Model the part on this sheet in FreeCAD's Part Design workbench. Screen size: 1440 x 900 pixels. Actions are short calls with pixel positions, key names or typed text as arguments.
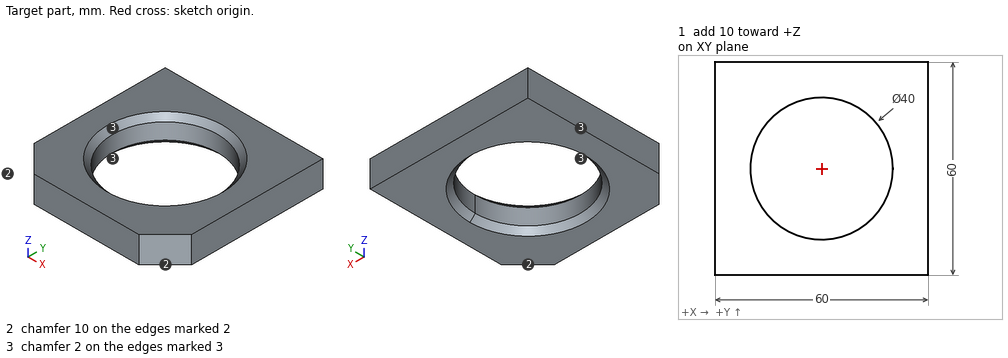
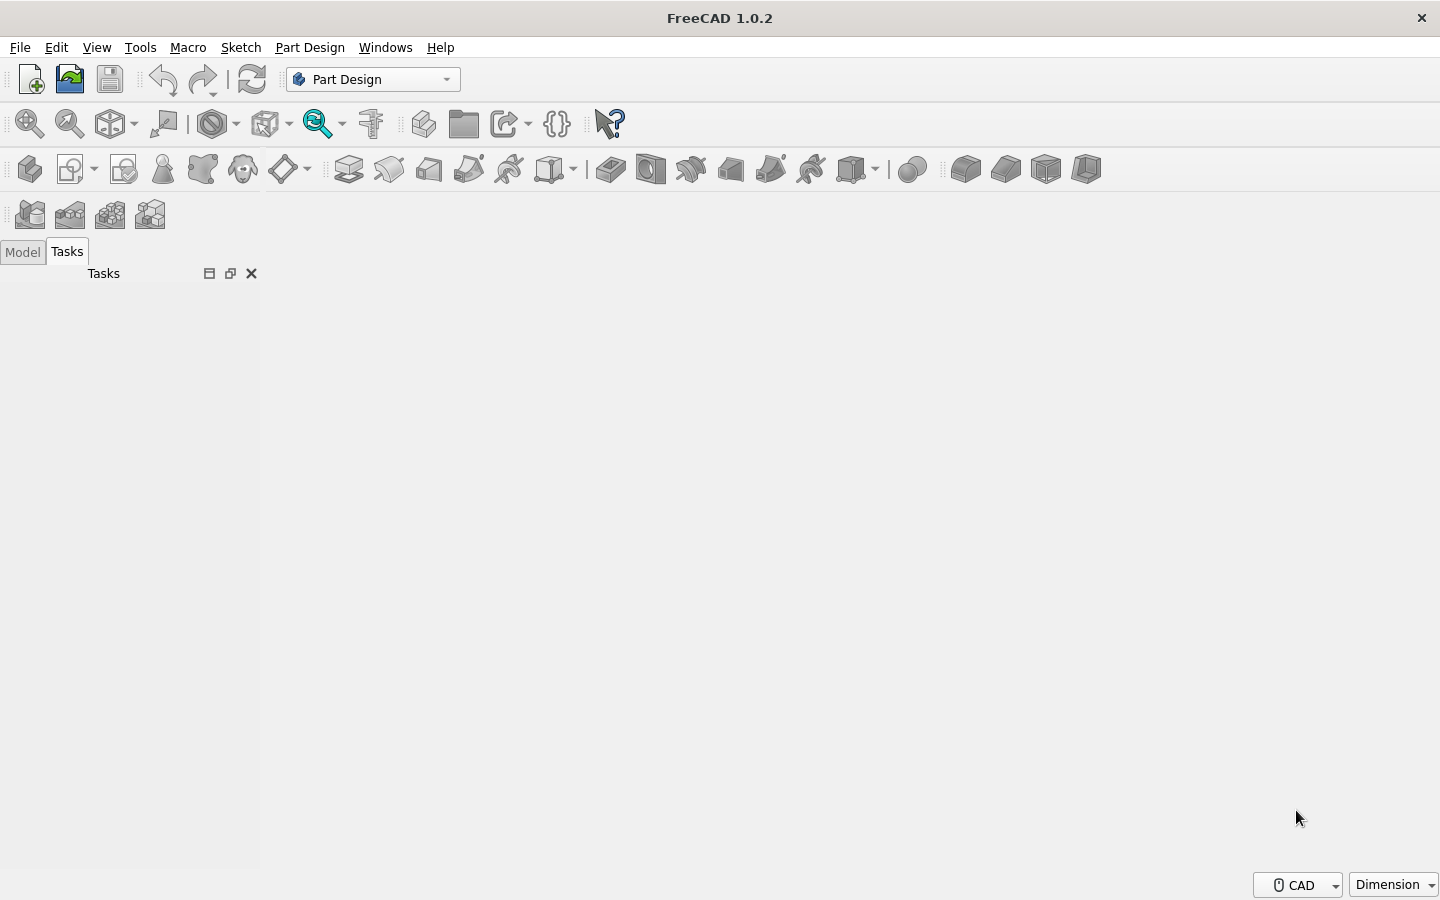
click(584, 80)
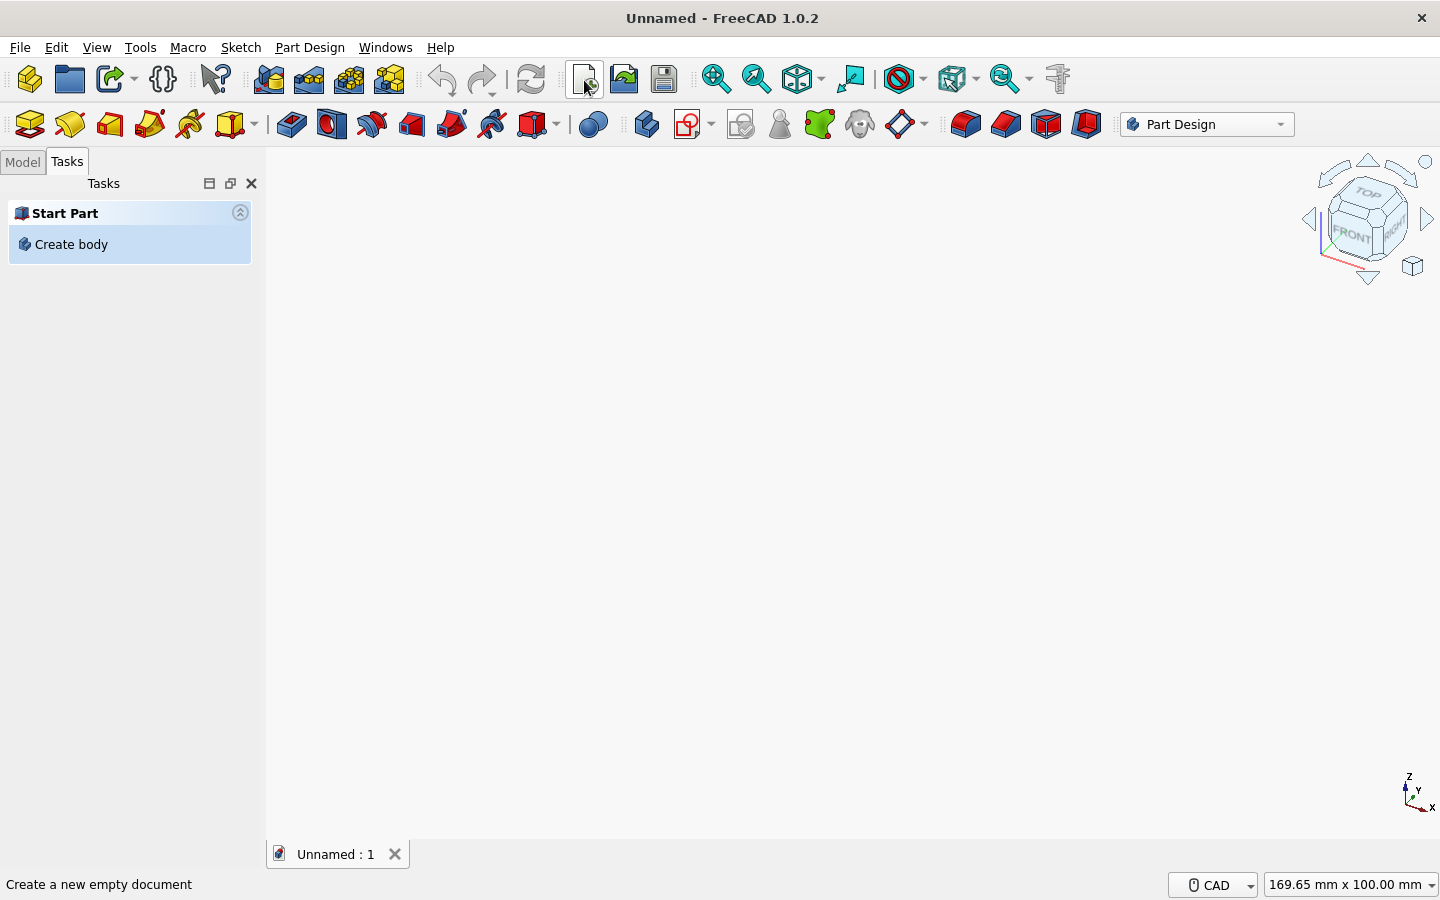
click(688, 124)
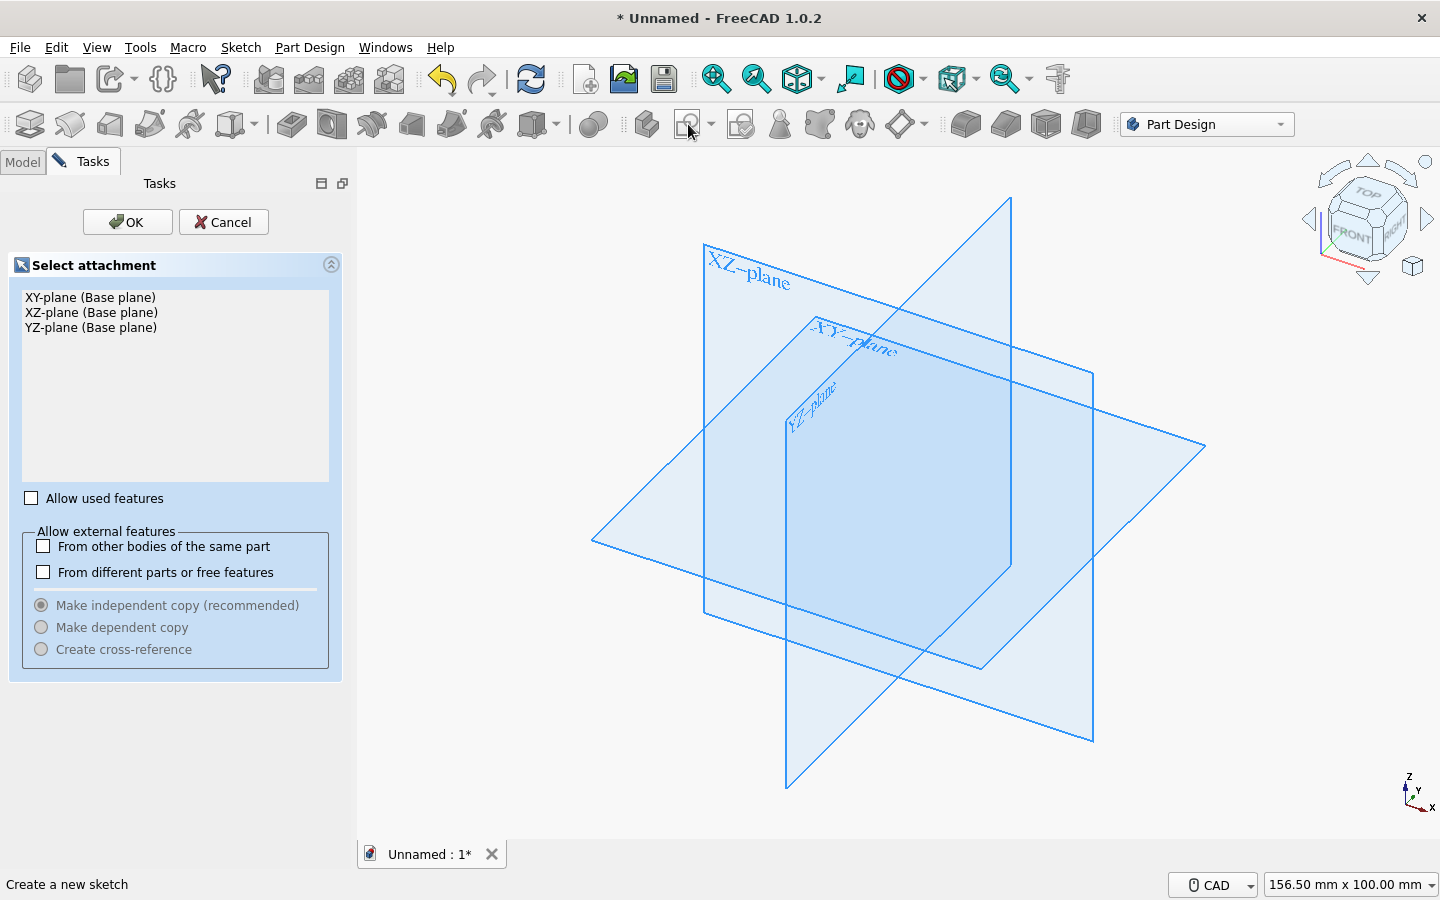
click(82, 298)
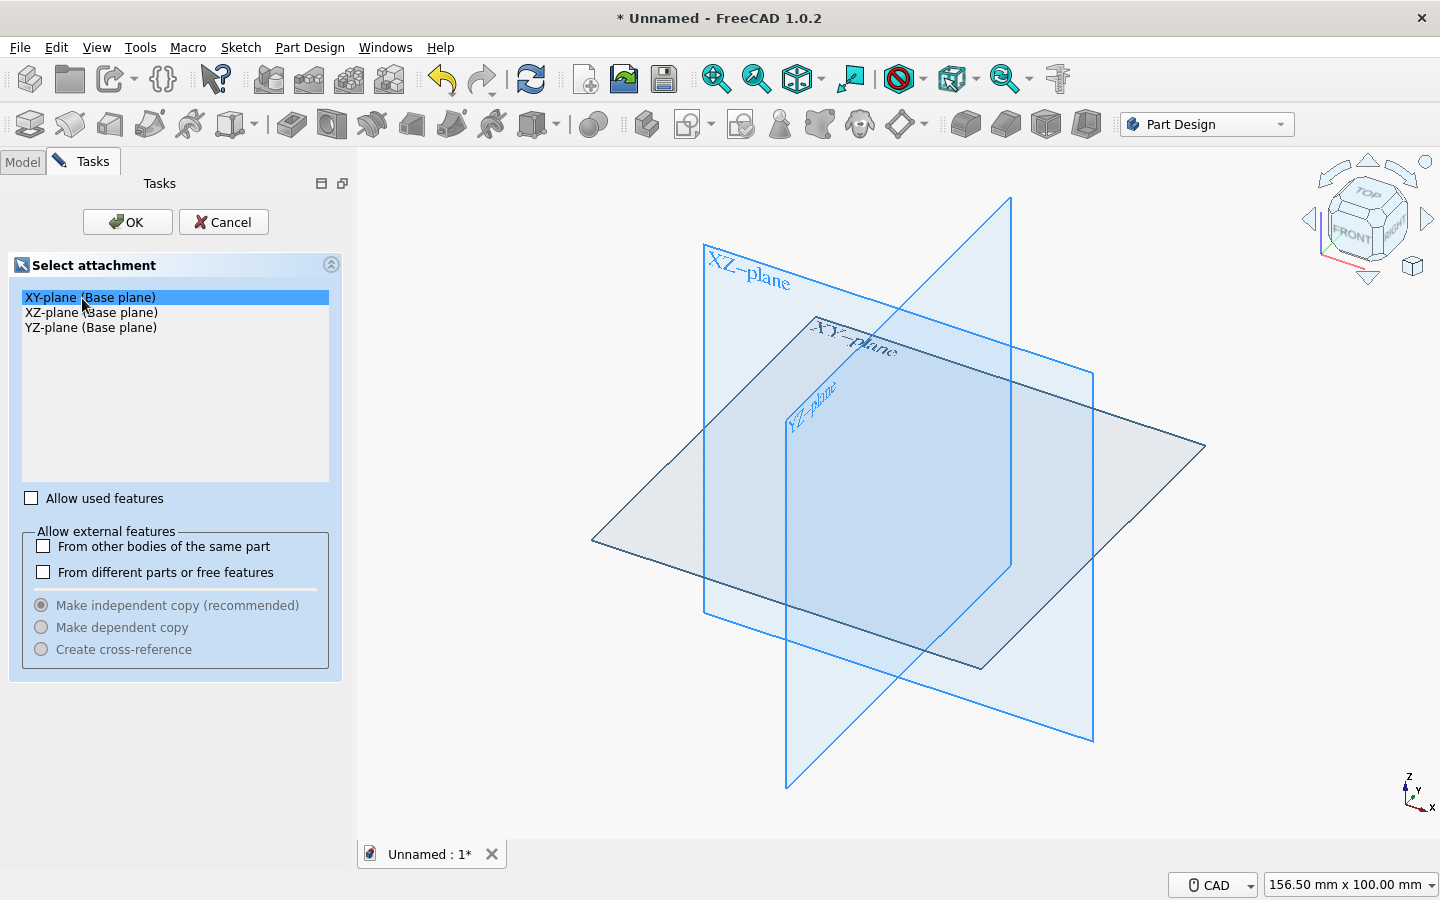
click(128, 222)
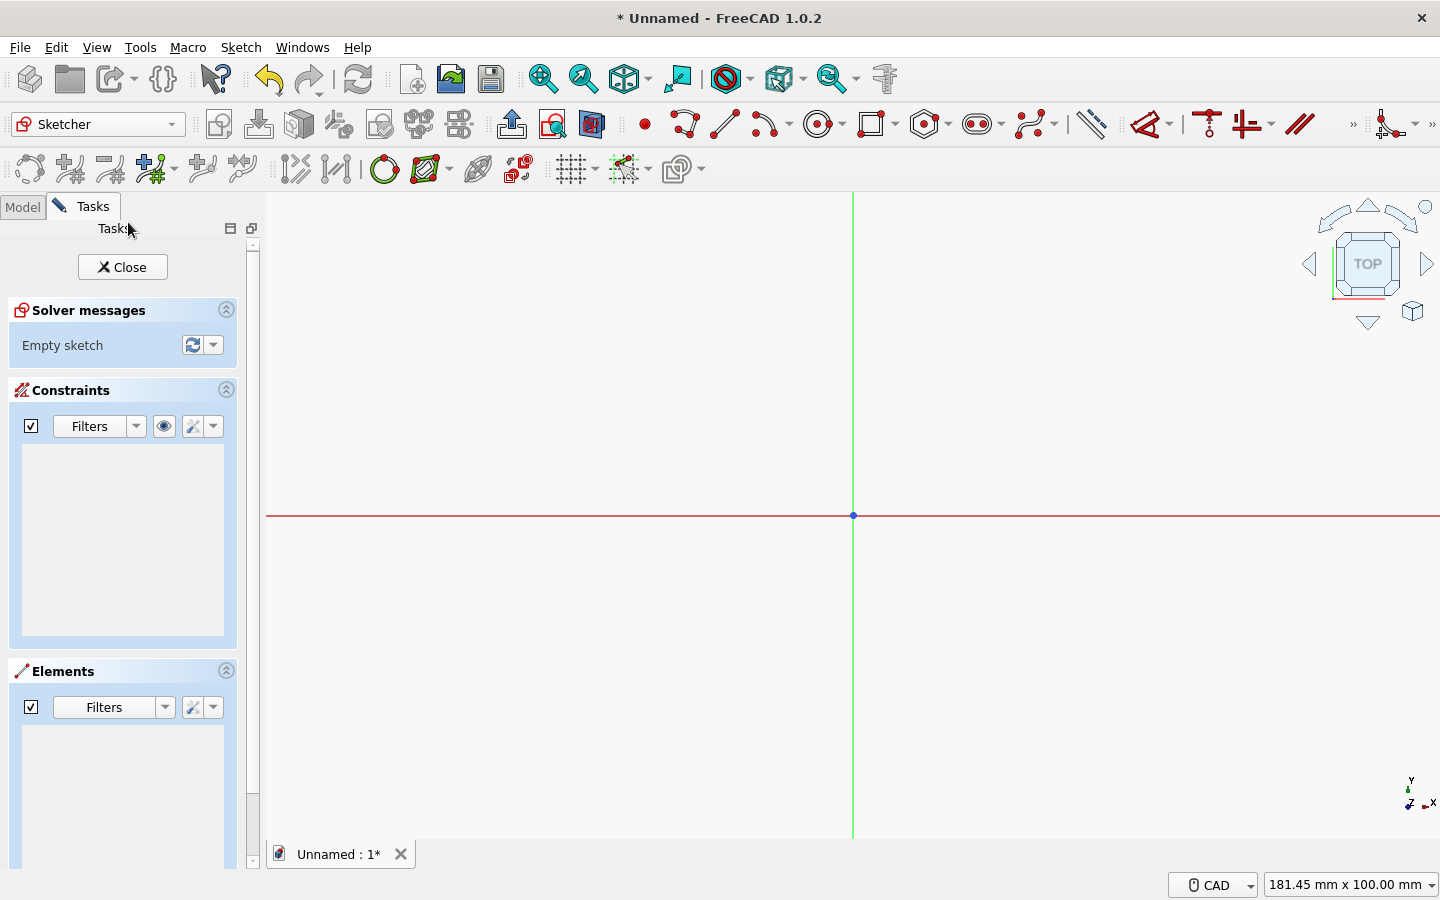
key(g)
key(v)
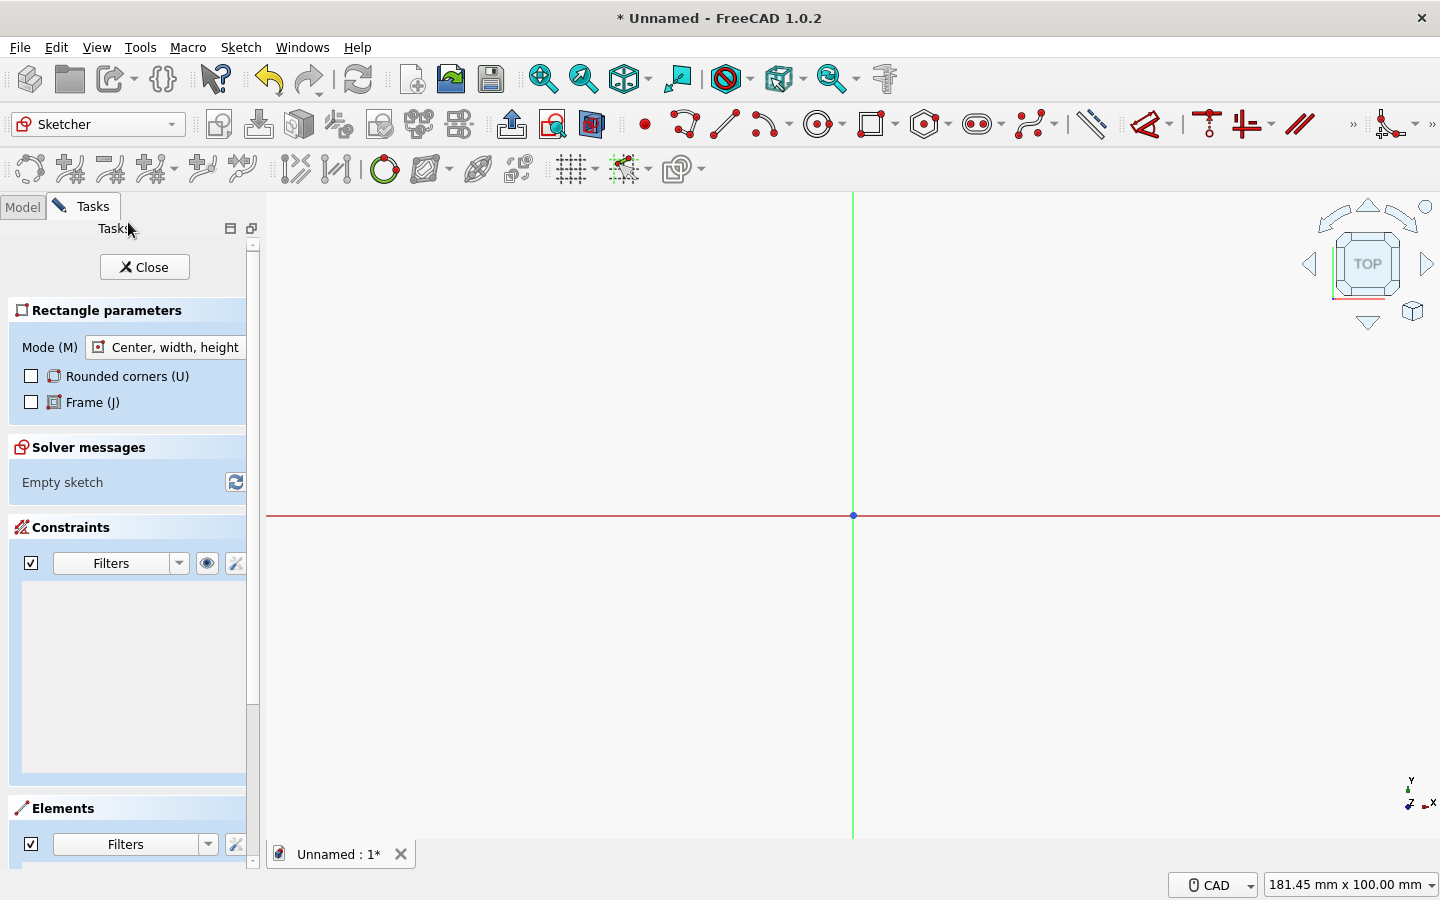
click(853, 516)
move(1047, 321)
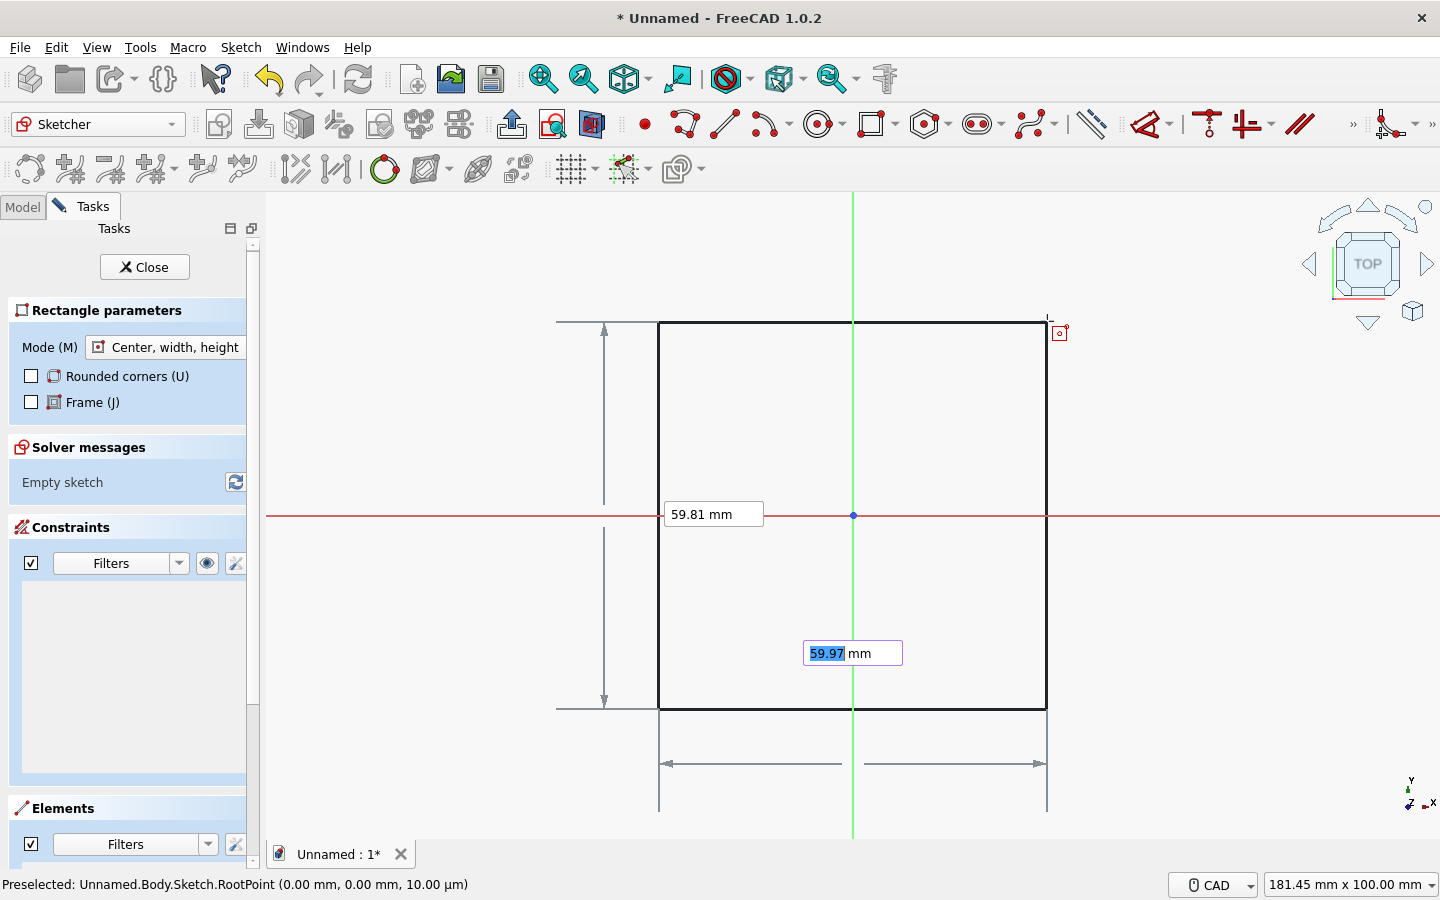
text(60)
key(Tab)
text(60)
key(Return)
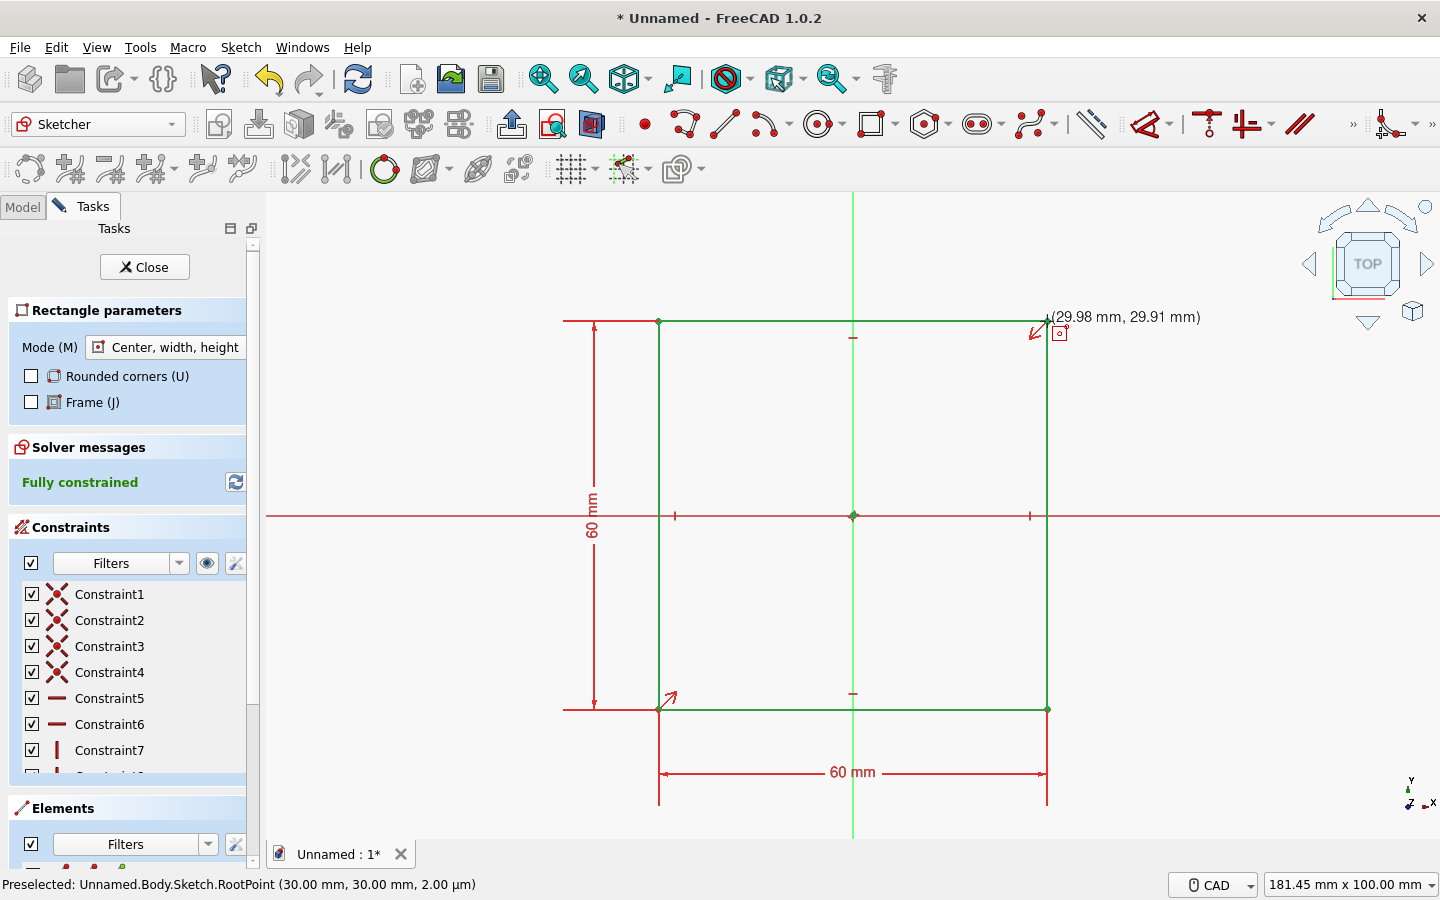
click(818, 124)